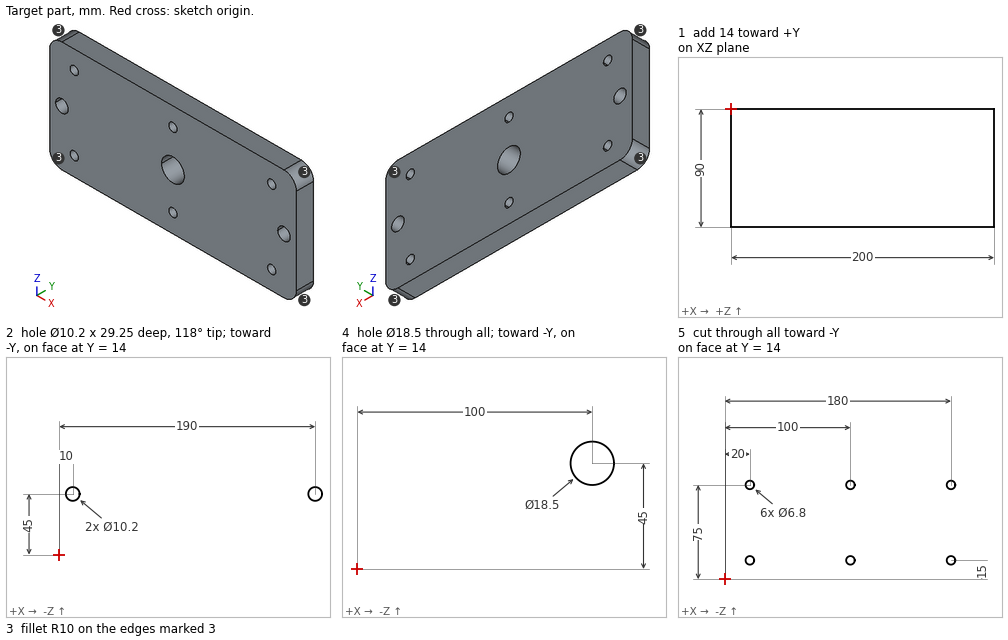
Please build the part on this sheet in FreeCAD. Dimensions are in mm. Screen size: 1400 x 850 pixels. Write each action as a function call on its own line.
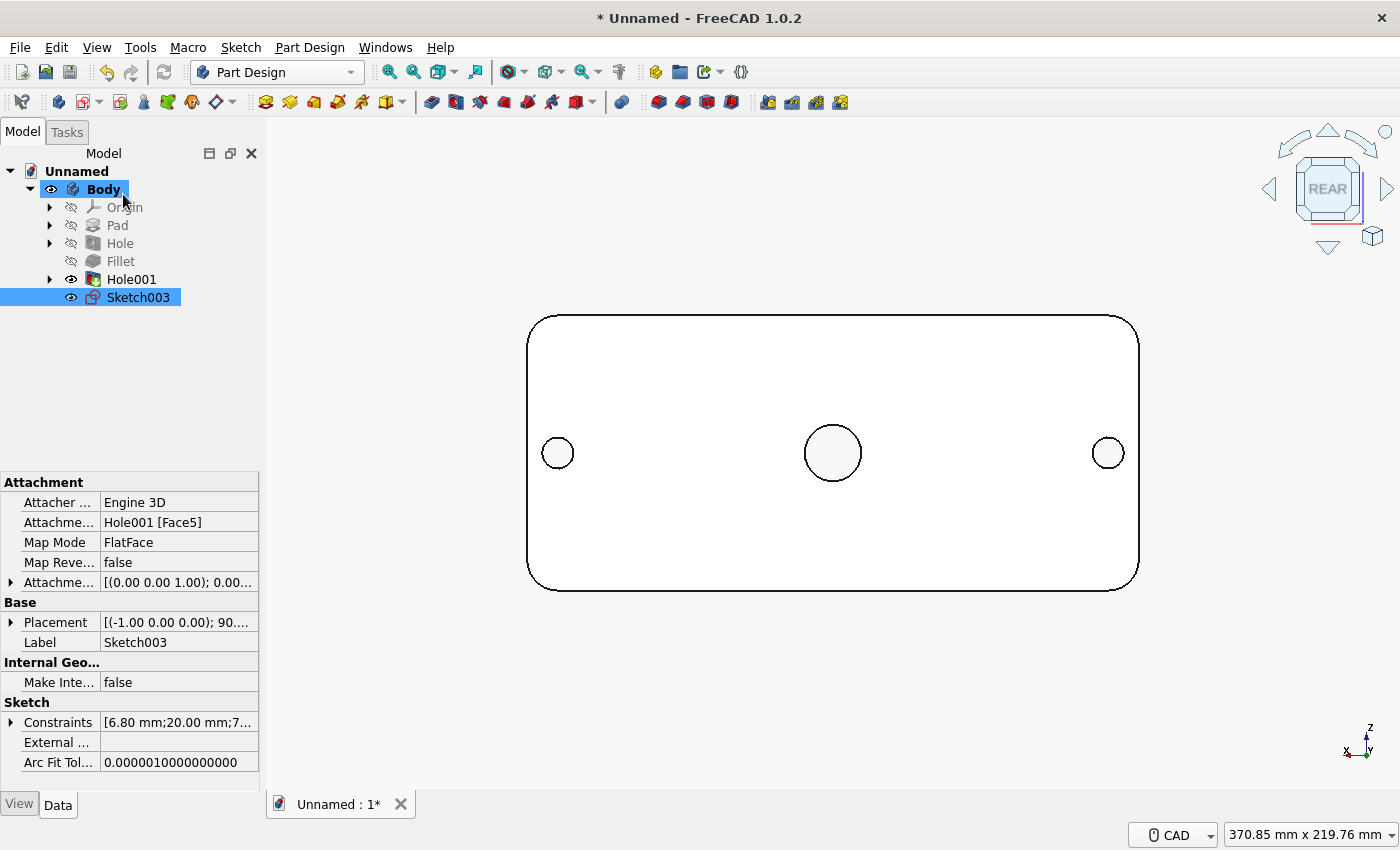
click(432, 102)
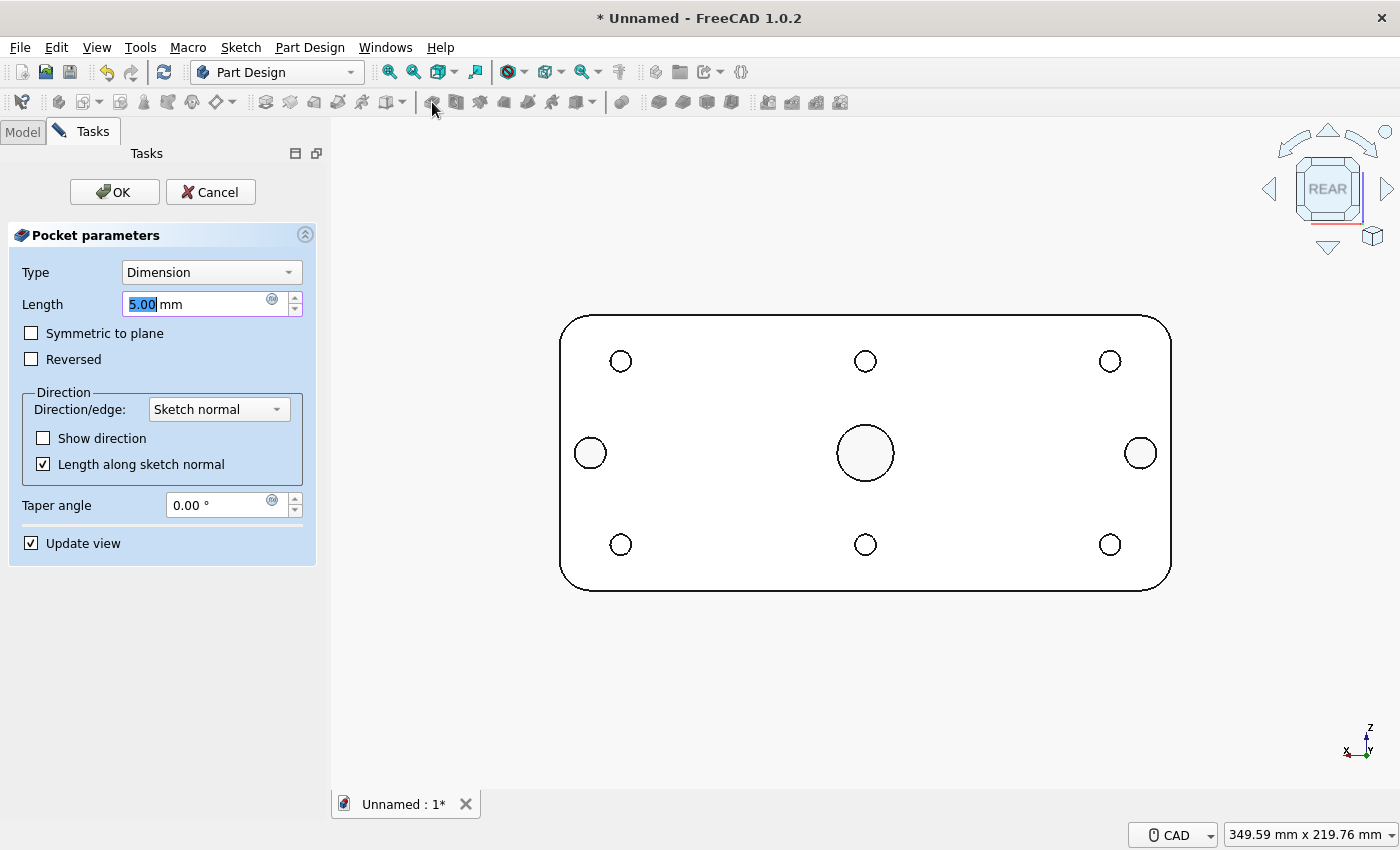
click(212, 272)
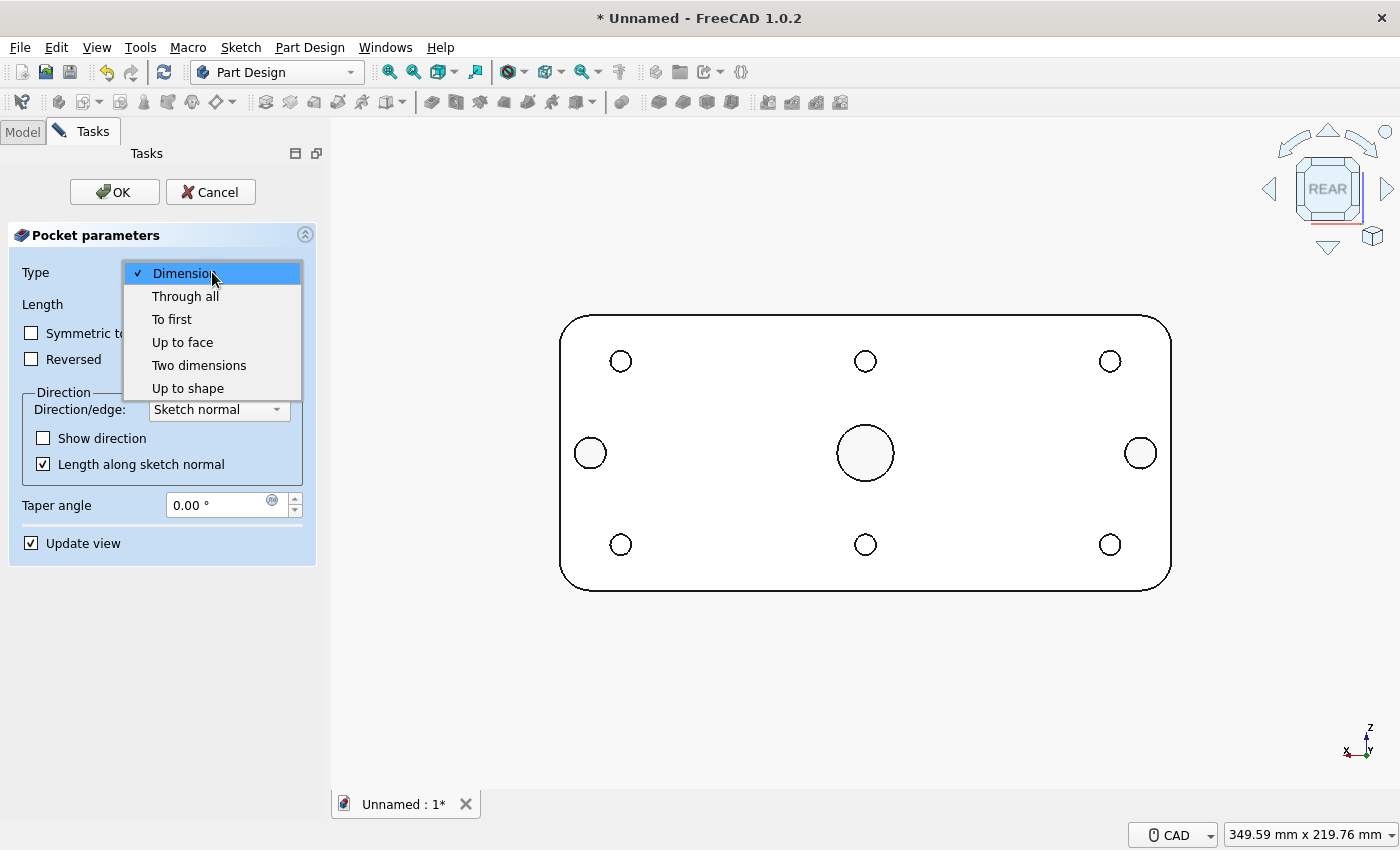
click(212, 296)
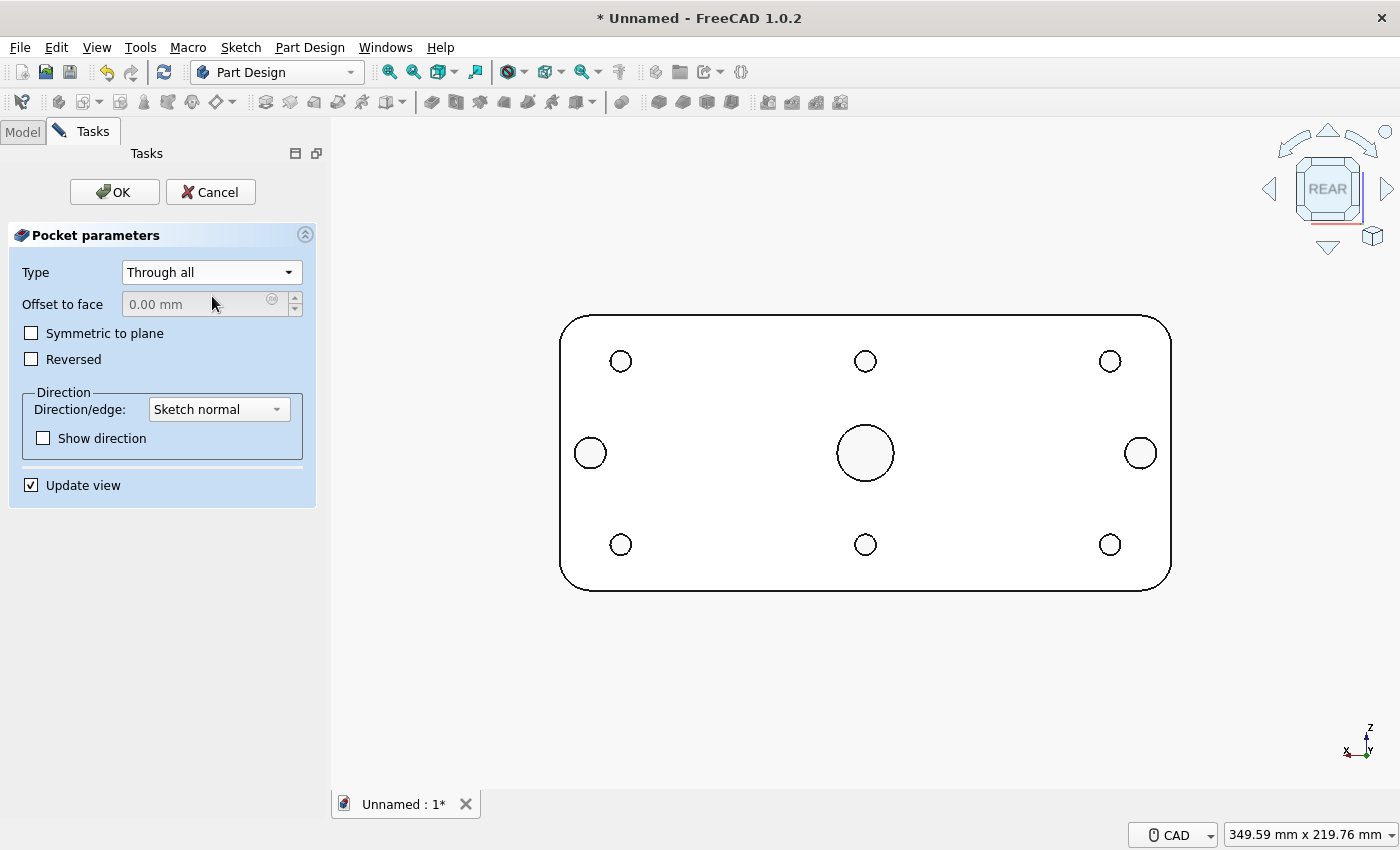
click(115, 192)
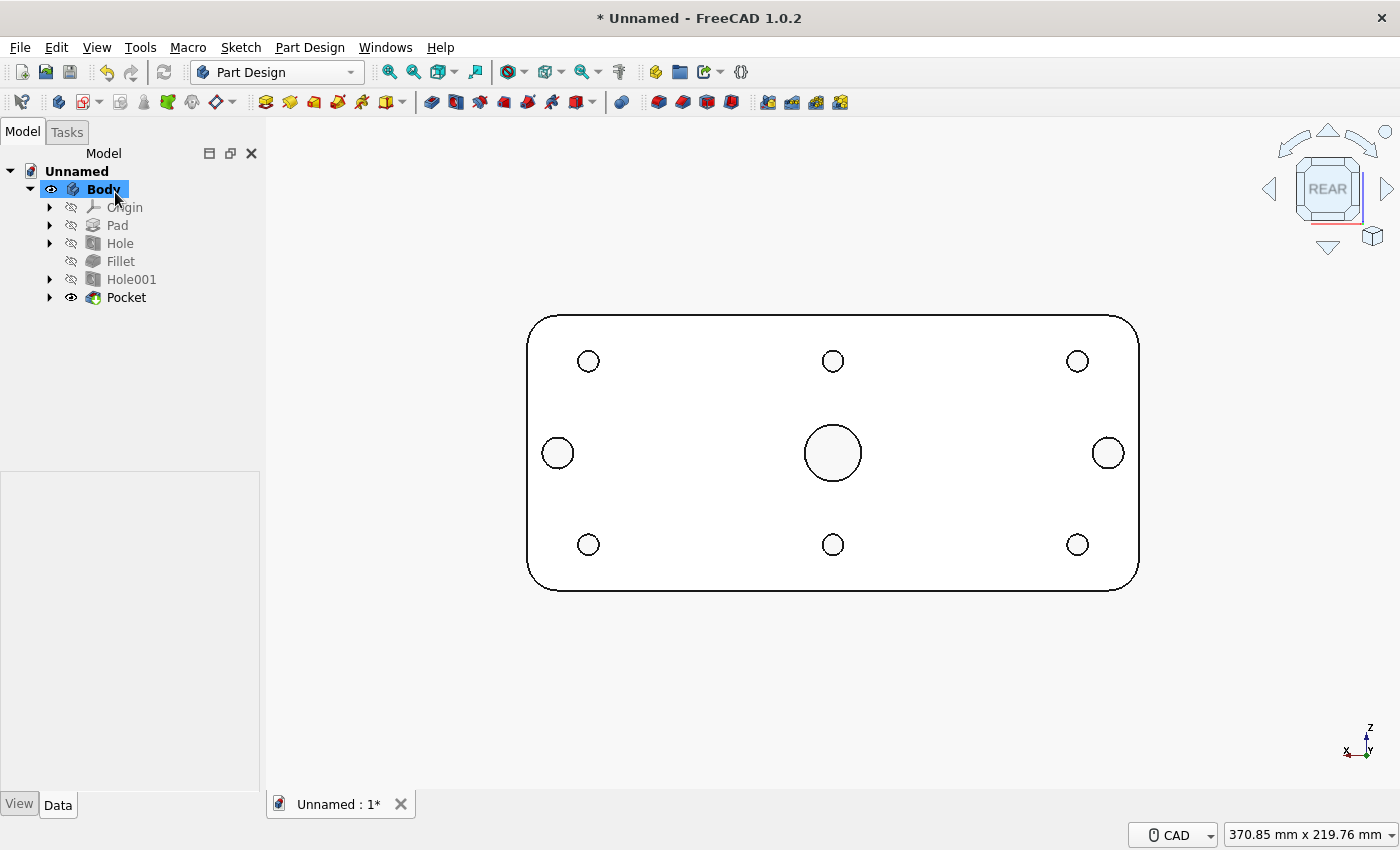
key(0)